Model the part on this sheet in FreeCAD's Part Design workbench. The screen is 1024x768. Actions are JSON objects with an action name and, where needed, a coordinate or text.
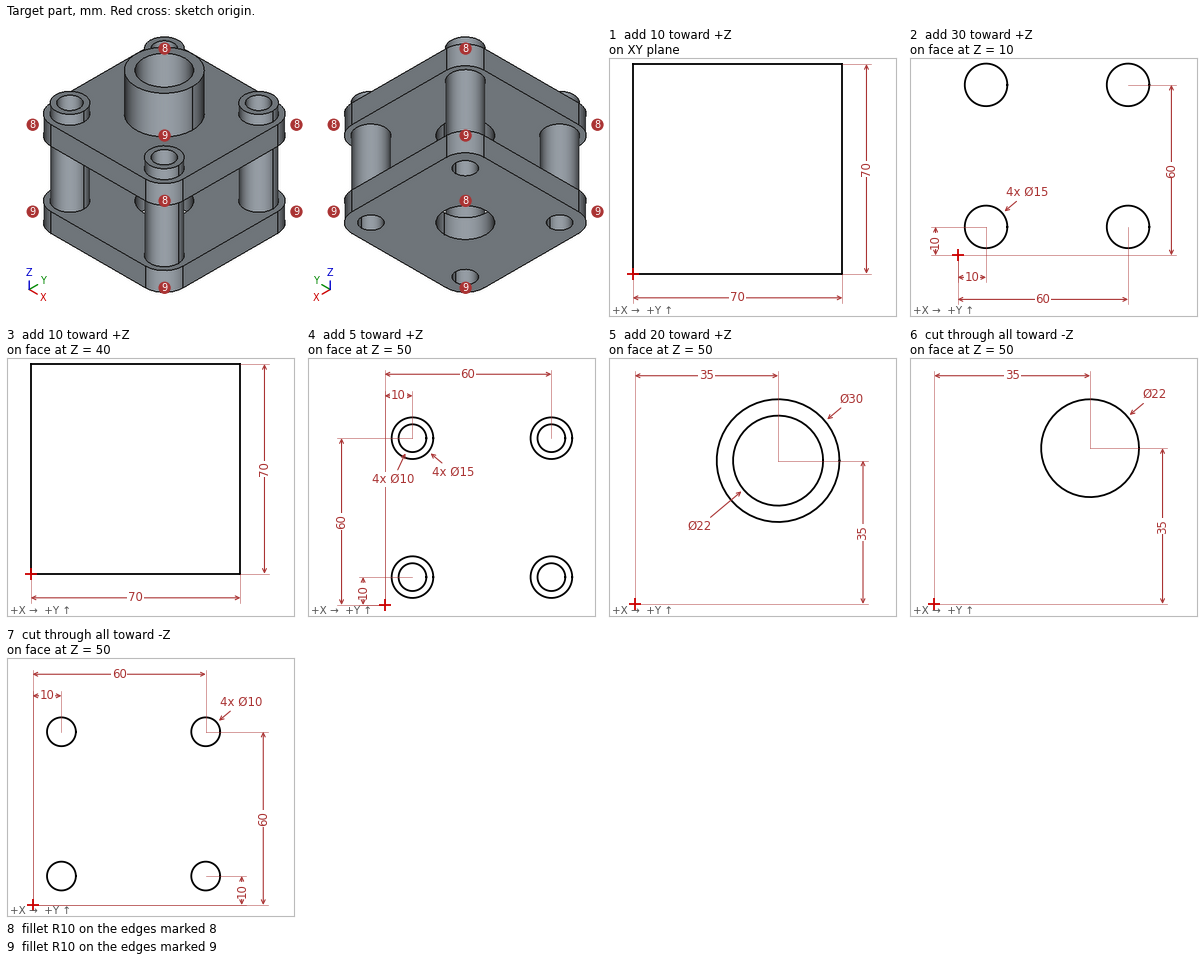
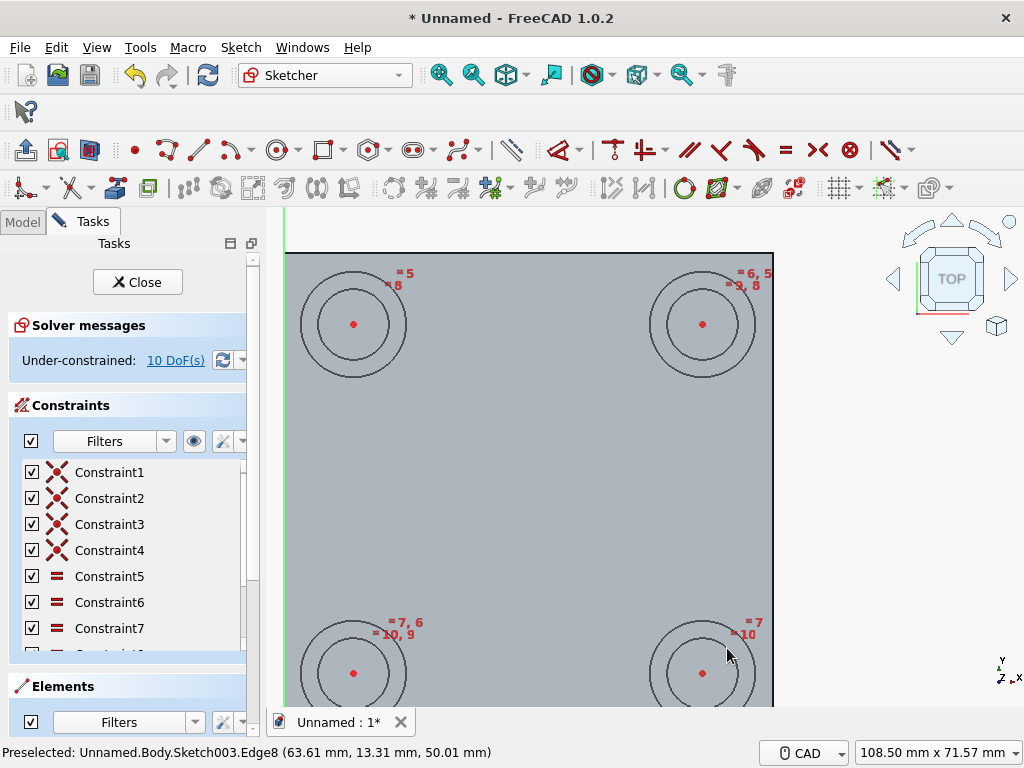
{"action": "left_click", "coordinate": [353, 324]}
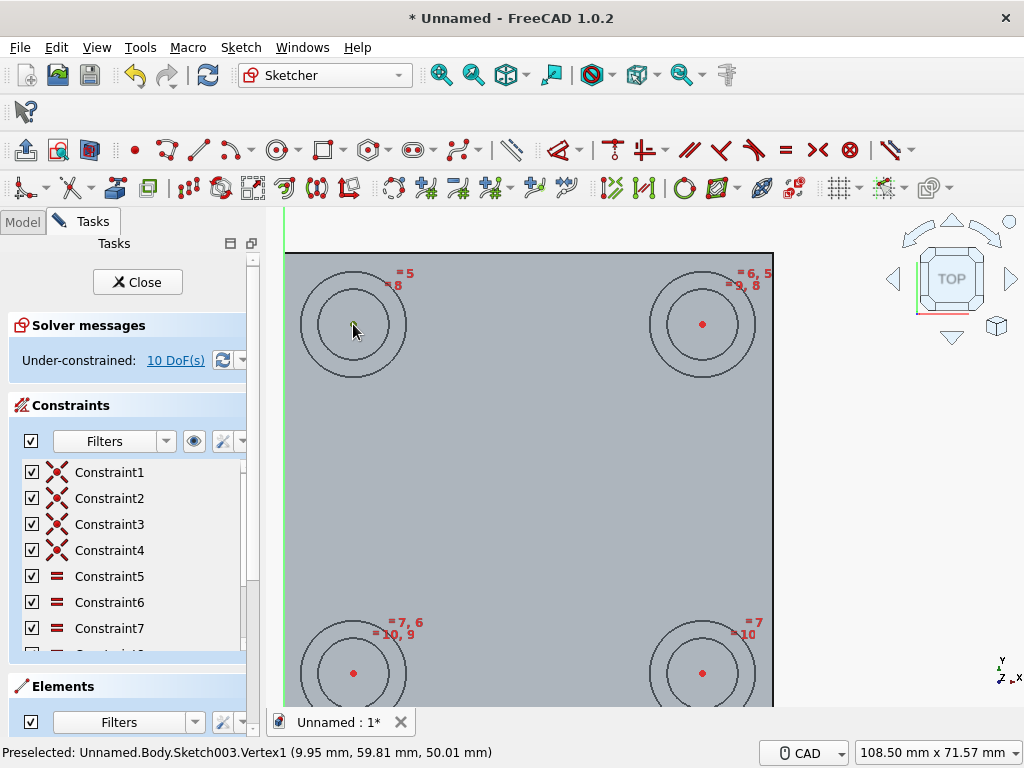
{"action": "left_click", "coordinate": [702, 324]}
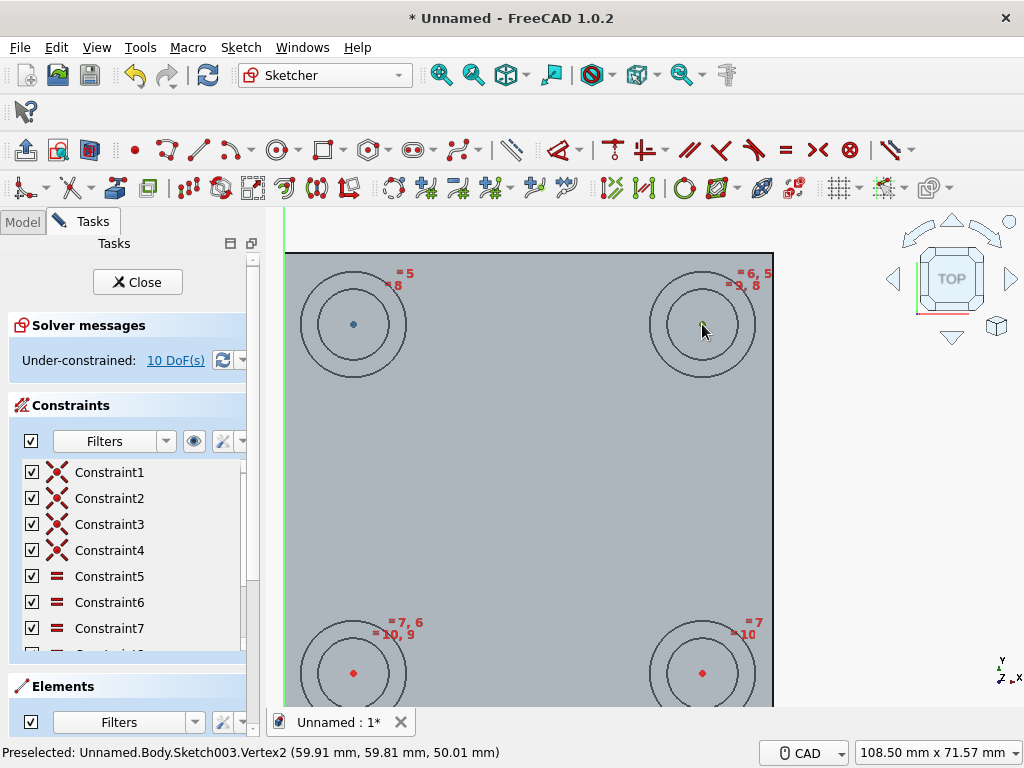
{"action": "key", "text": "h"}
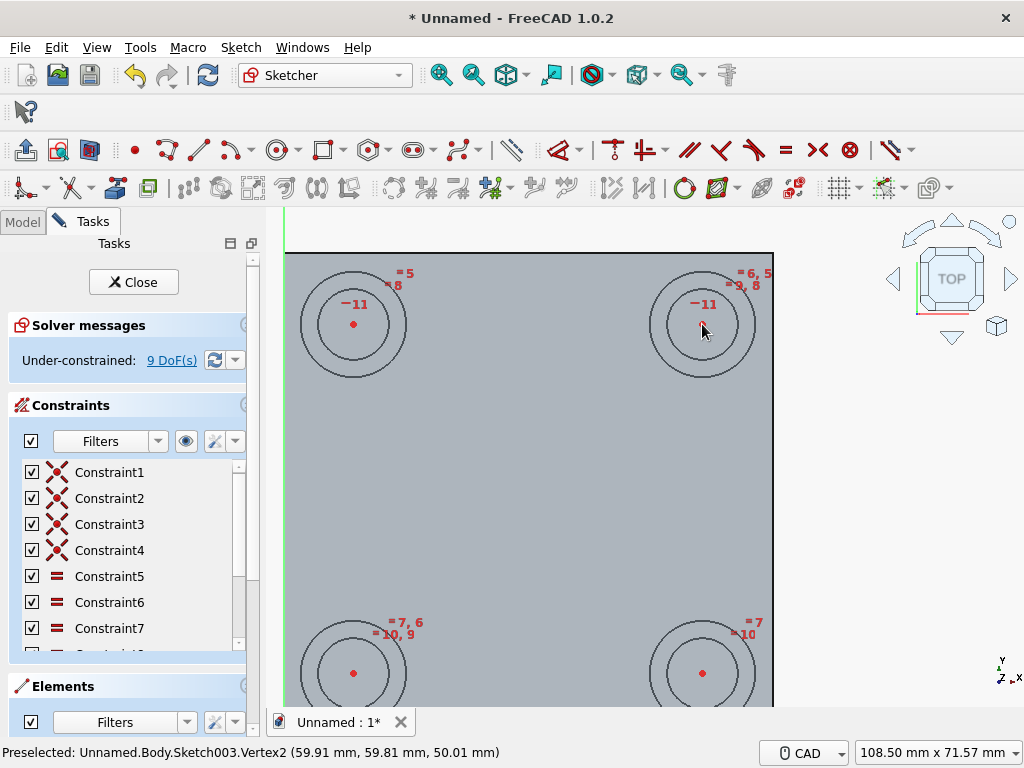
{"action": "left_click", "coordinate": [353, 324]}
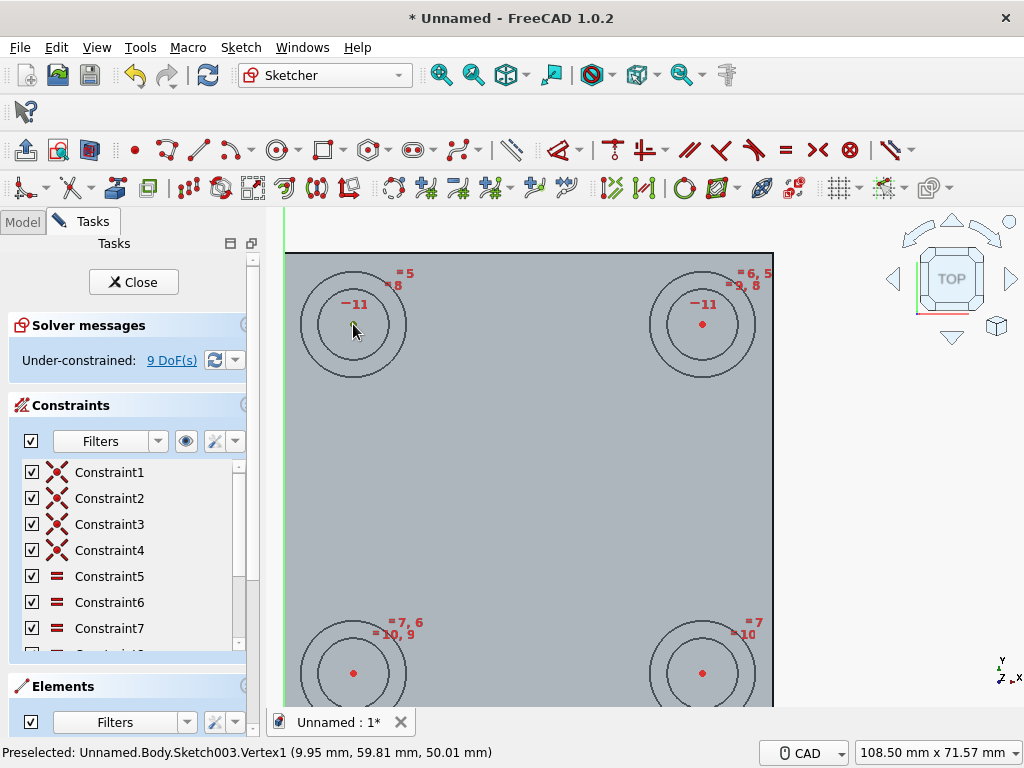
{"action": "left_click", "coordinate": [353, 674]}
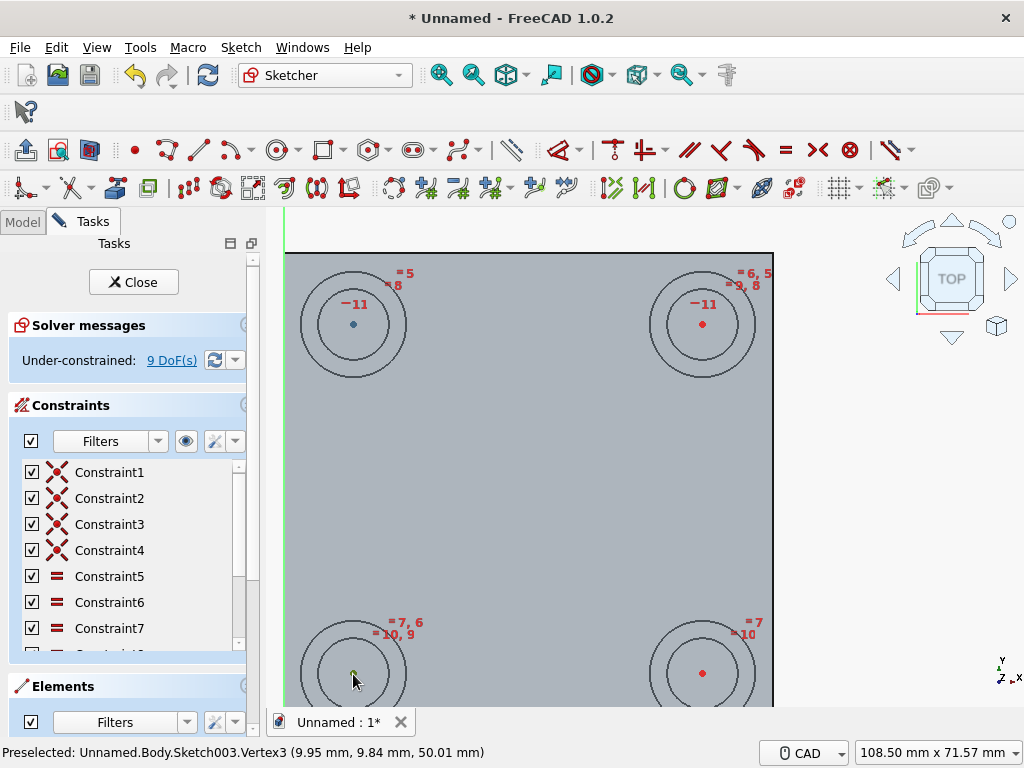
{"action": "key", "text": "v"}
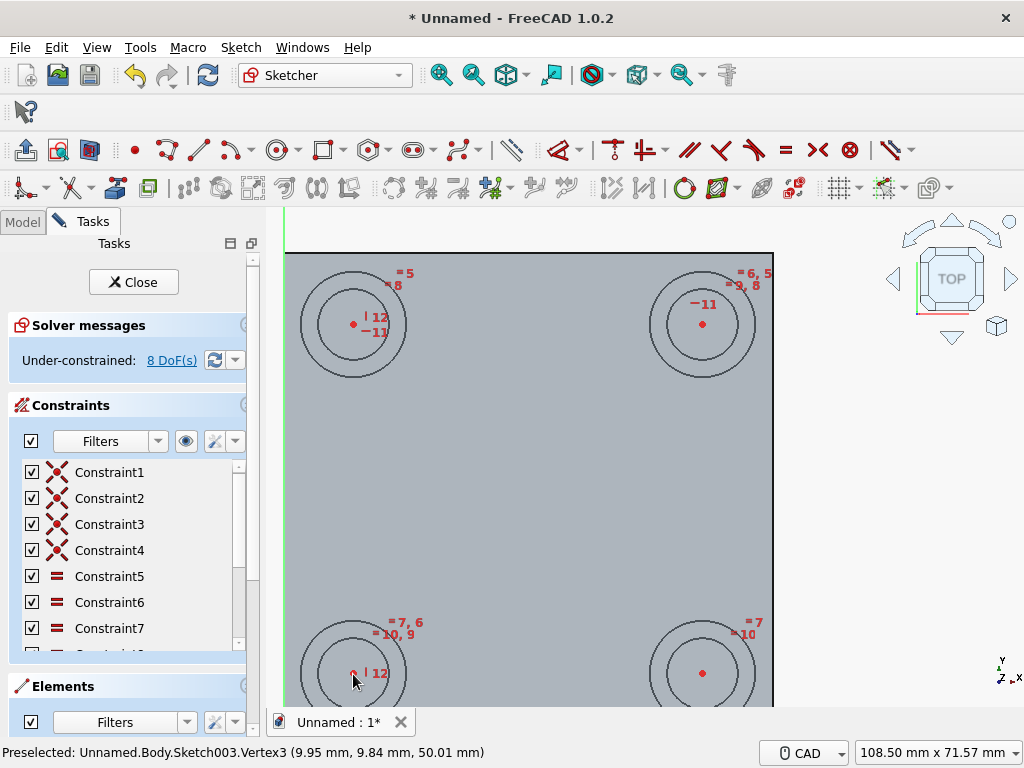
{"action": "left_click", "coordinate": [702, 324]}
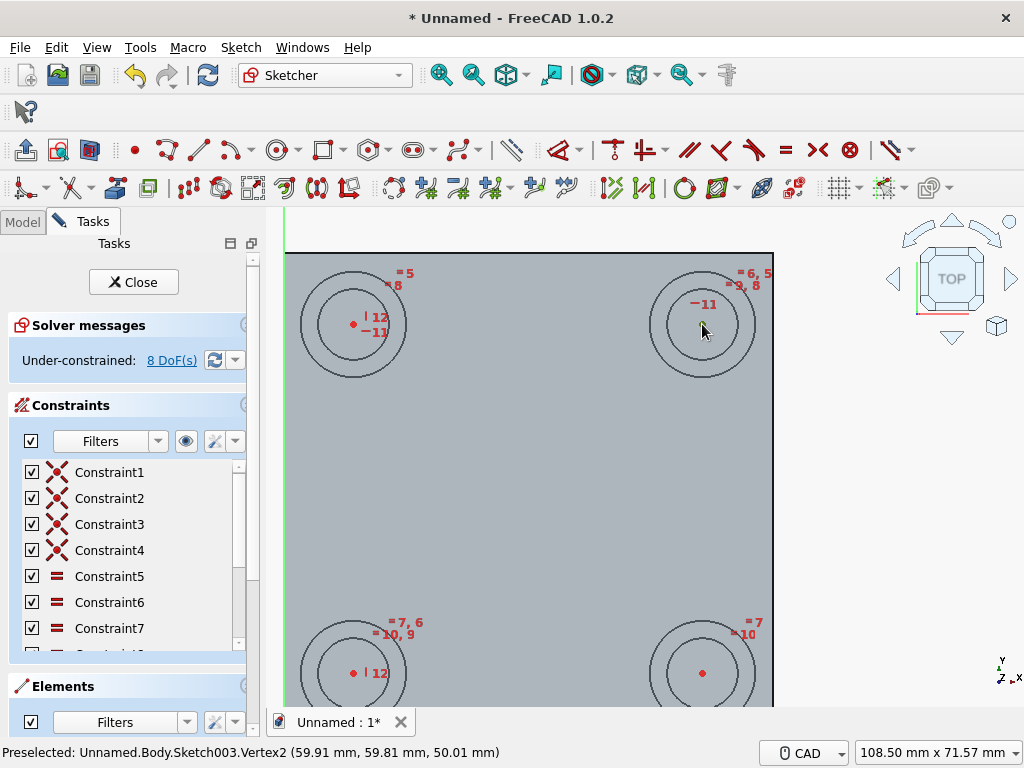
{"action": "left_click", "coordinate": [702, 674]}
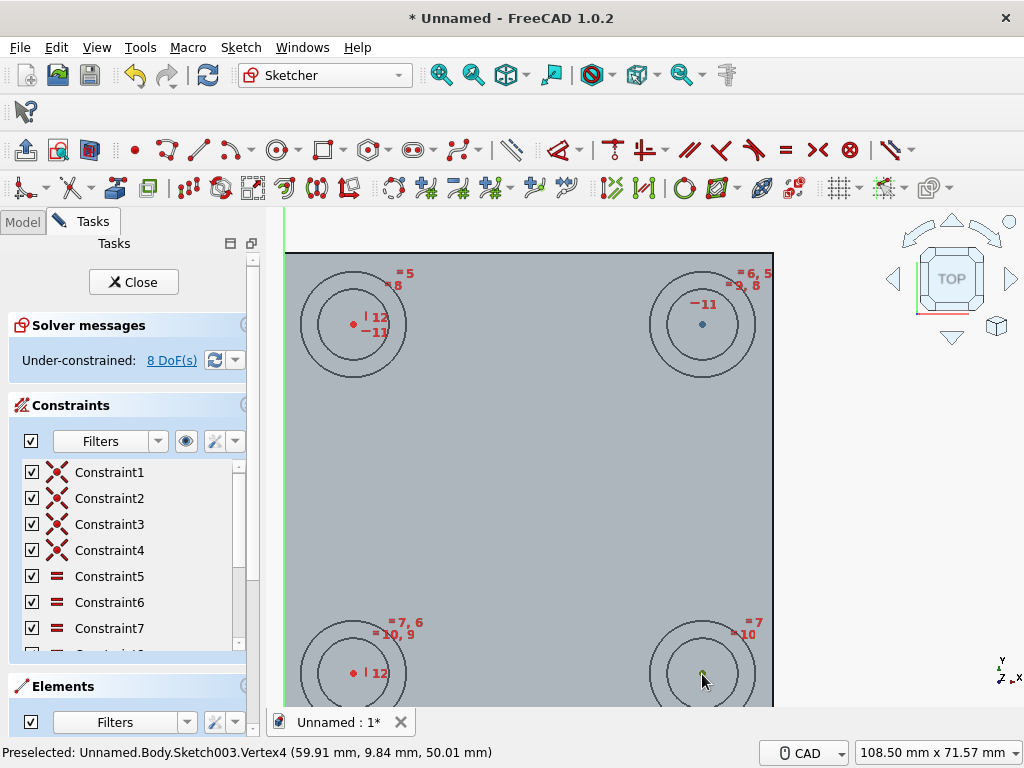
{"action": "key", "text": "v"}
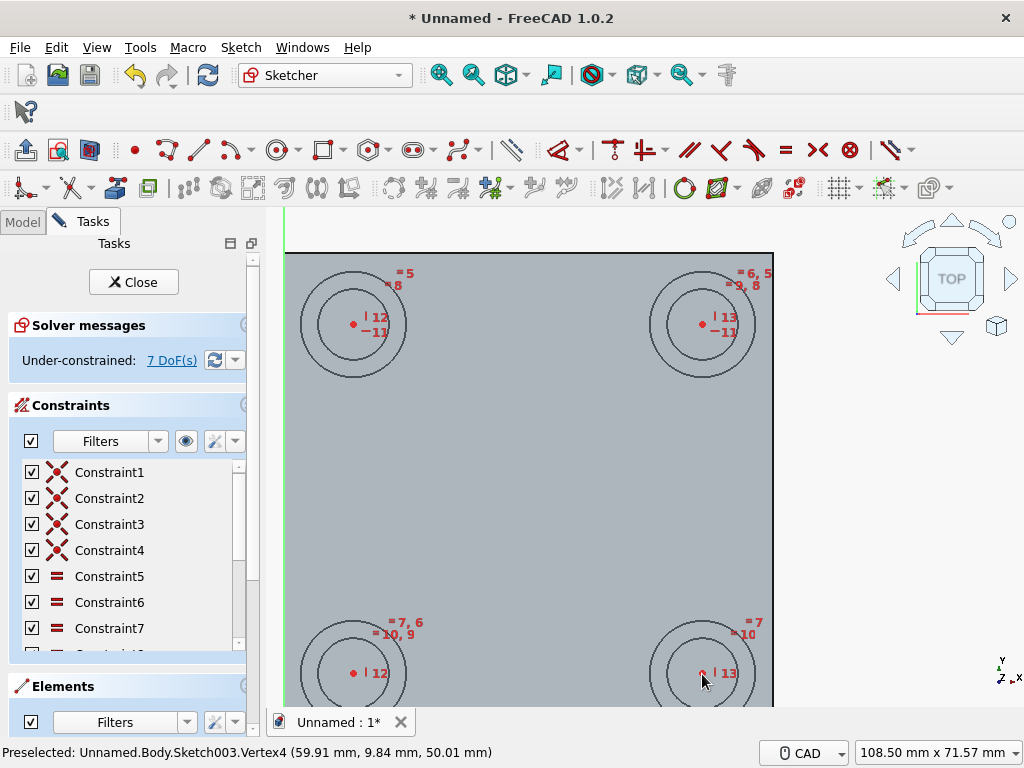
{"action": "left_click", "coordinate": [353, 674]}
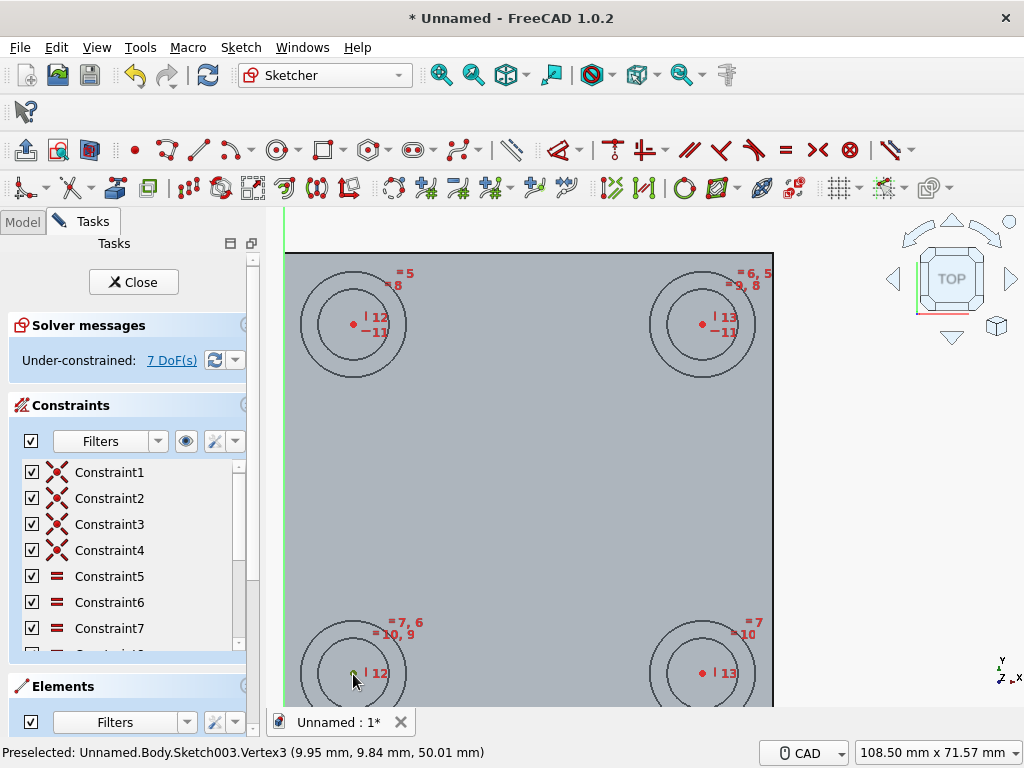
{"action": "left_click", "coordinate": [702, 674]}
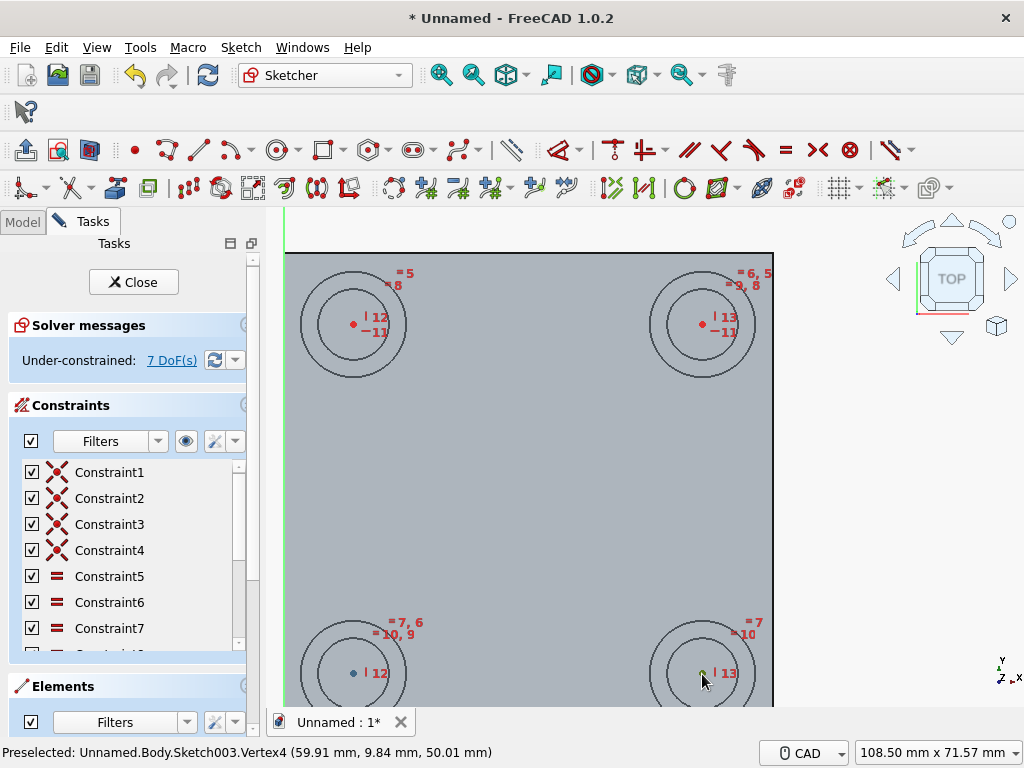
{"action": "left_click", "coordinate": [668, 150]}